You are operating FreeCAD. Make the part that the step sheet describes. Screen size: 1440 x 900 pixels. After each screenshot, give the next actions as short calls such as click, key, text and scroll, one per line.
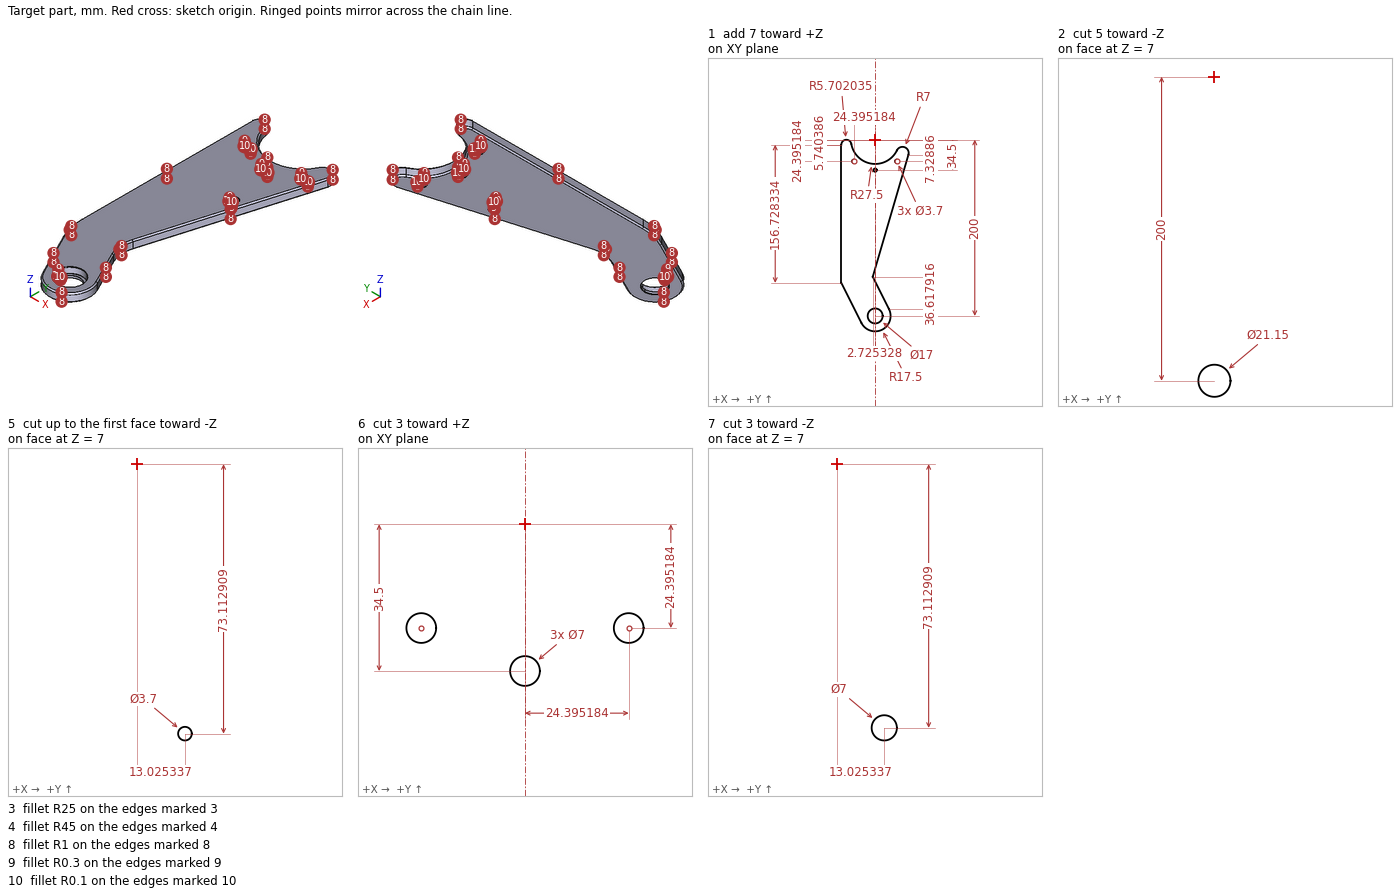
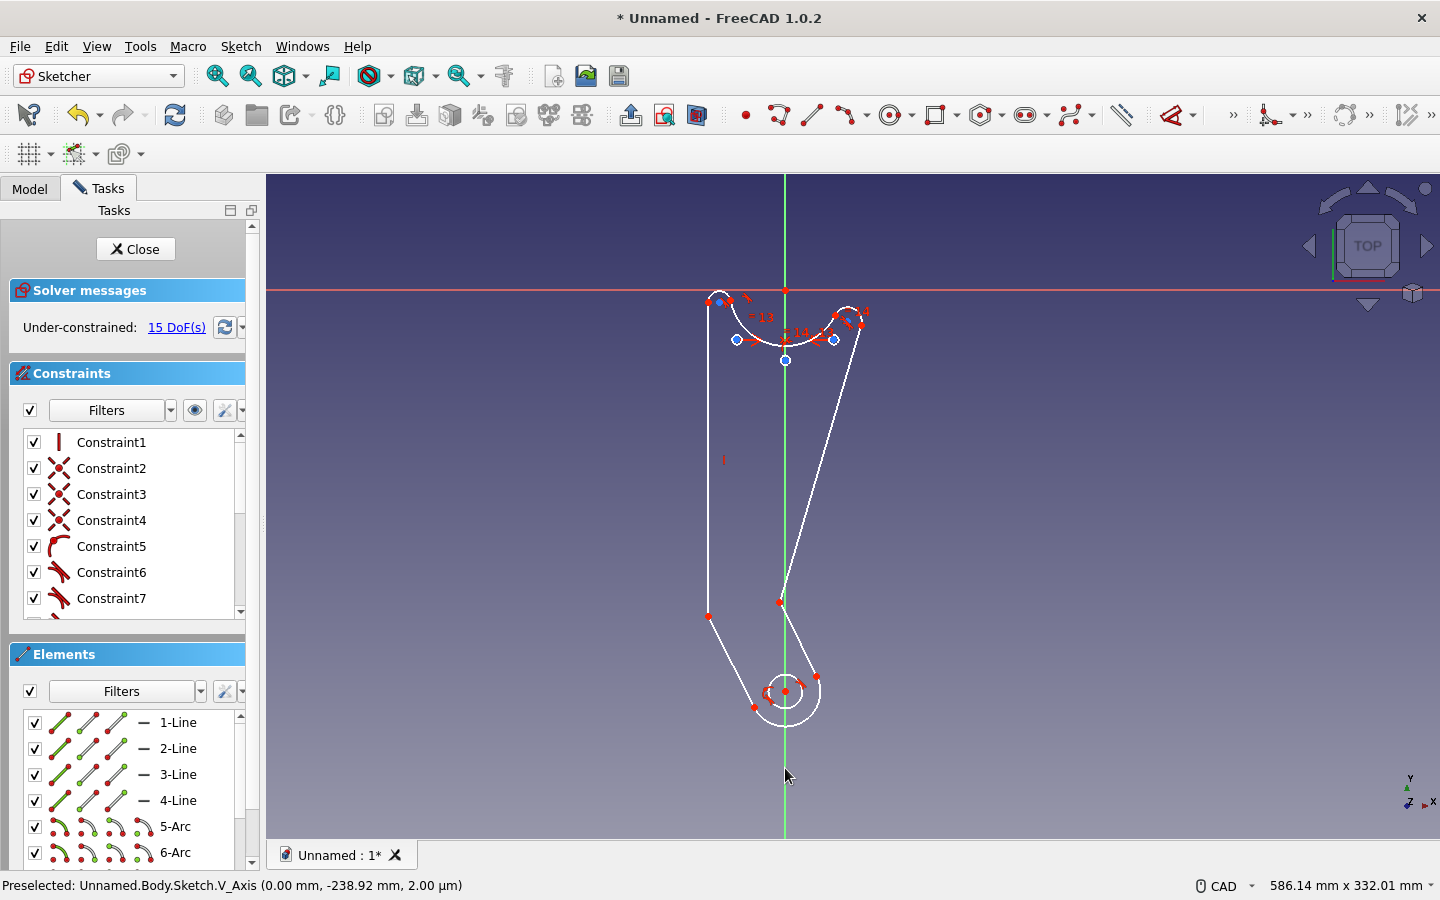
key(d)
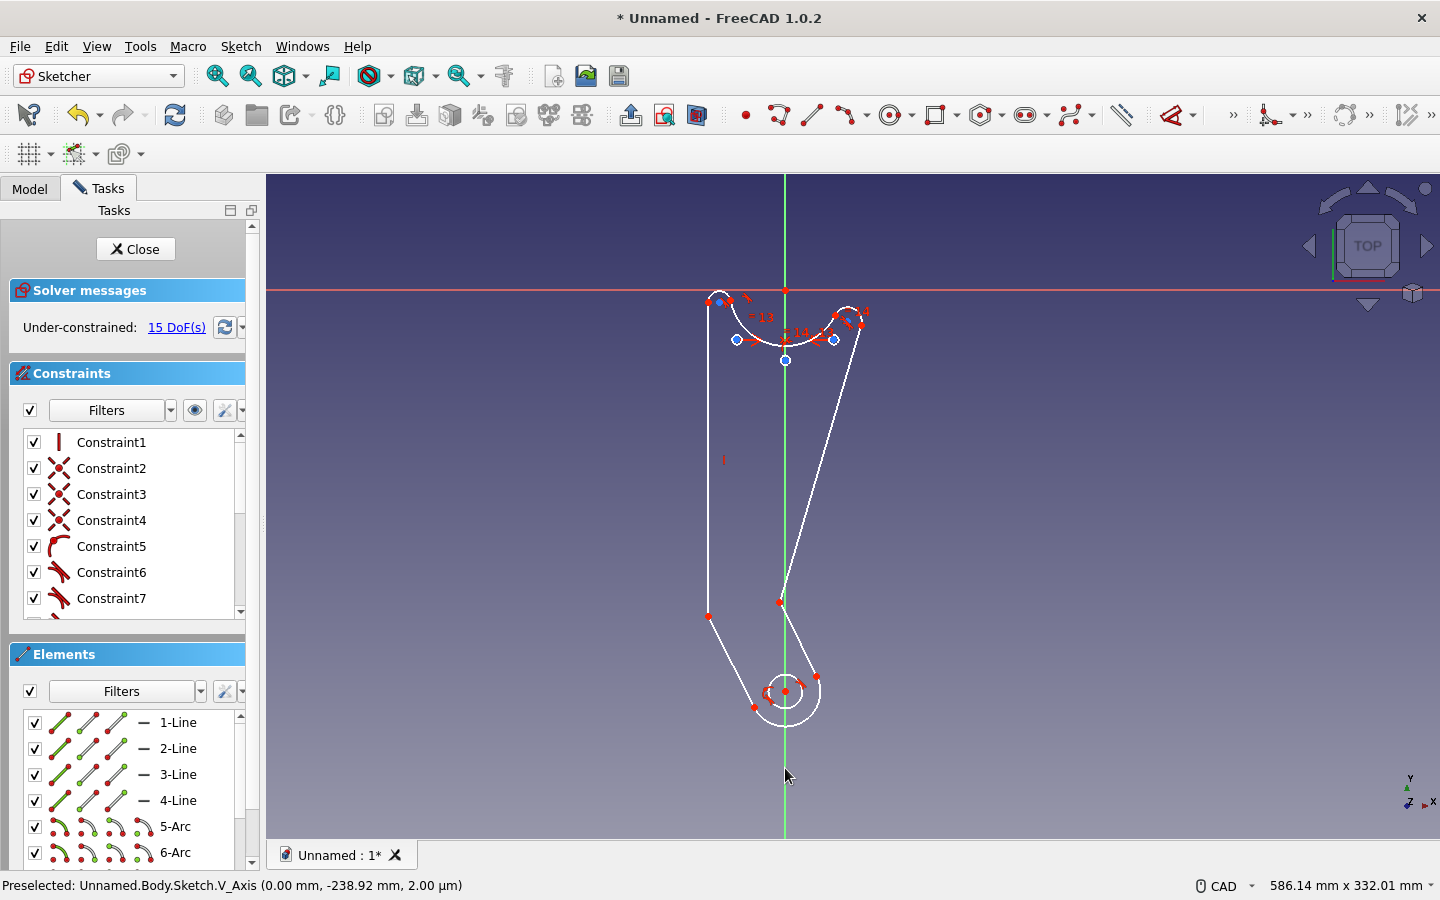
click(816, 708)
click(844, 723)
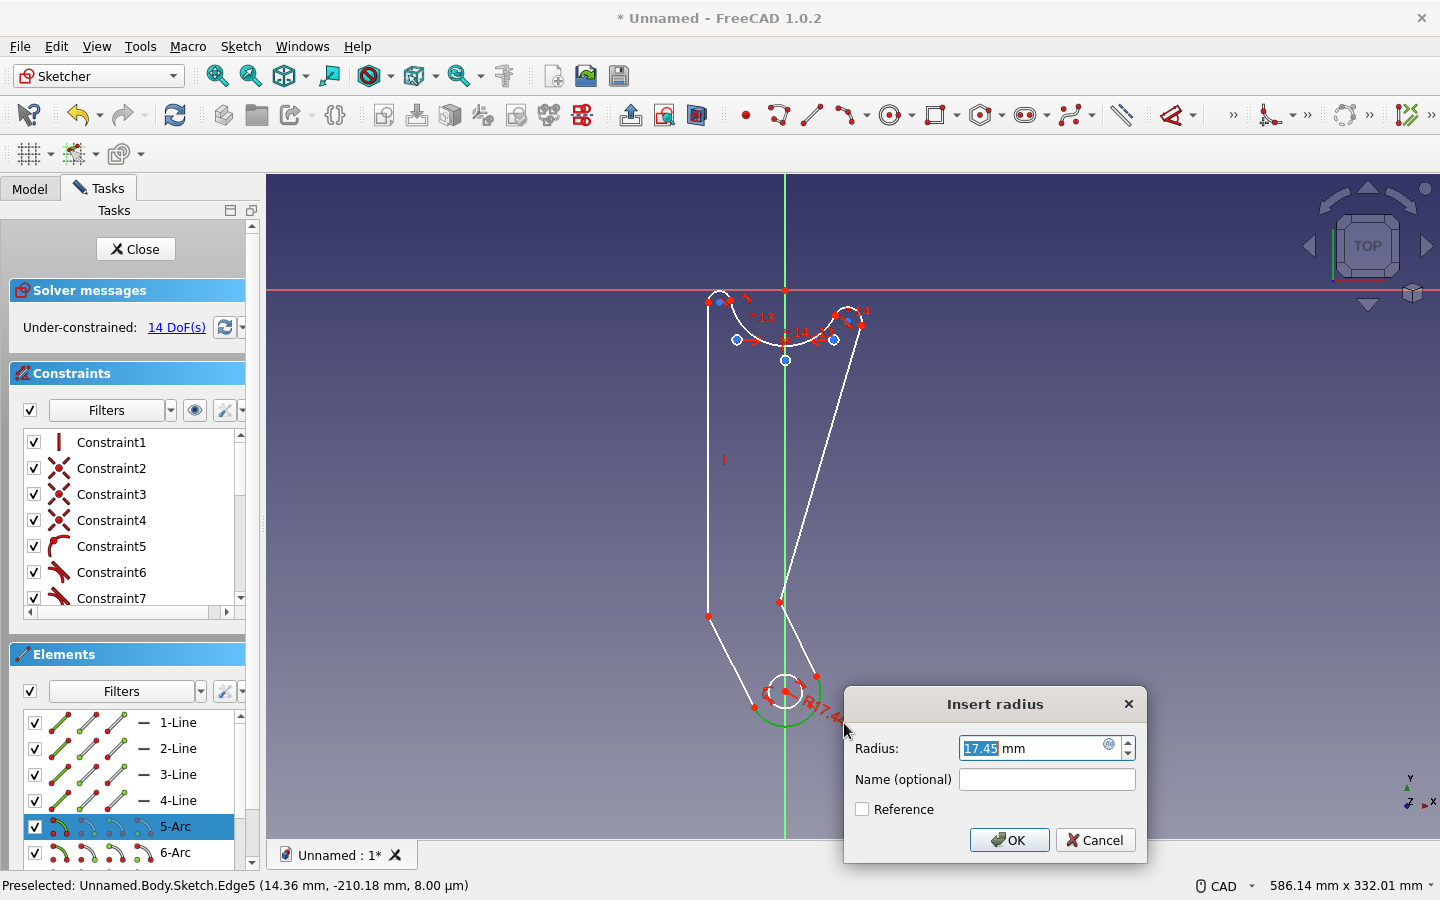
text(17.5)
key(Return)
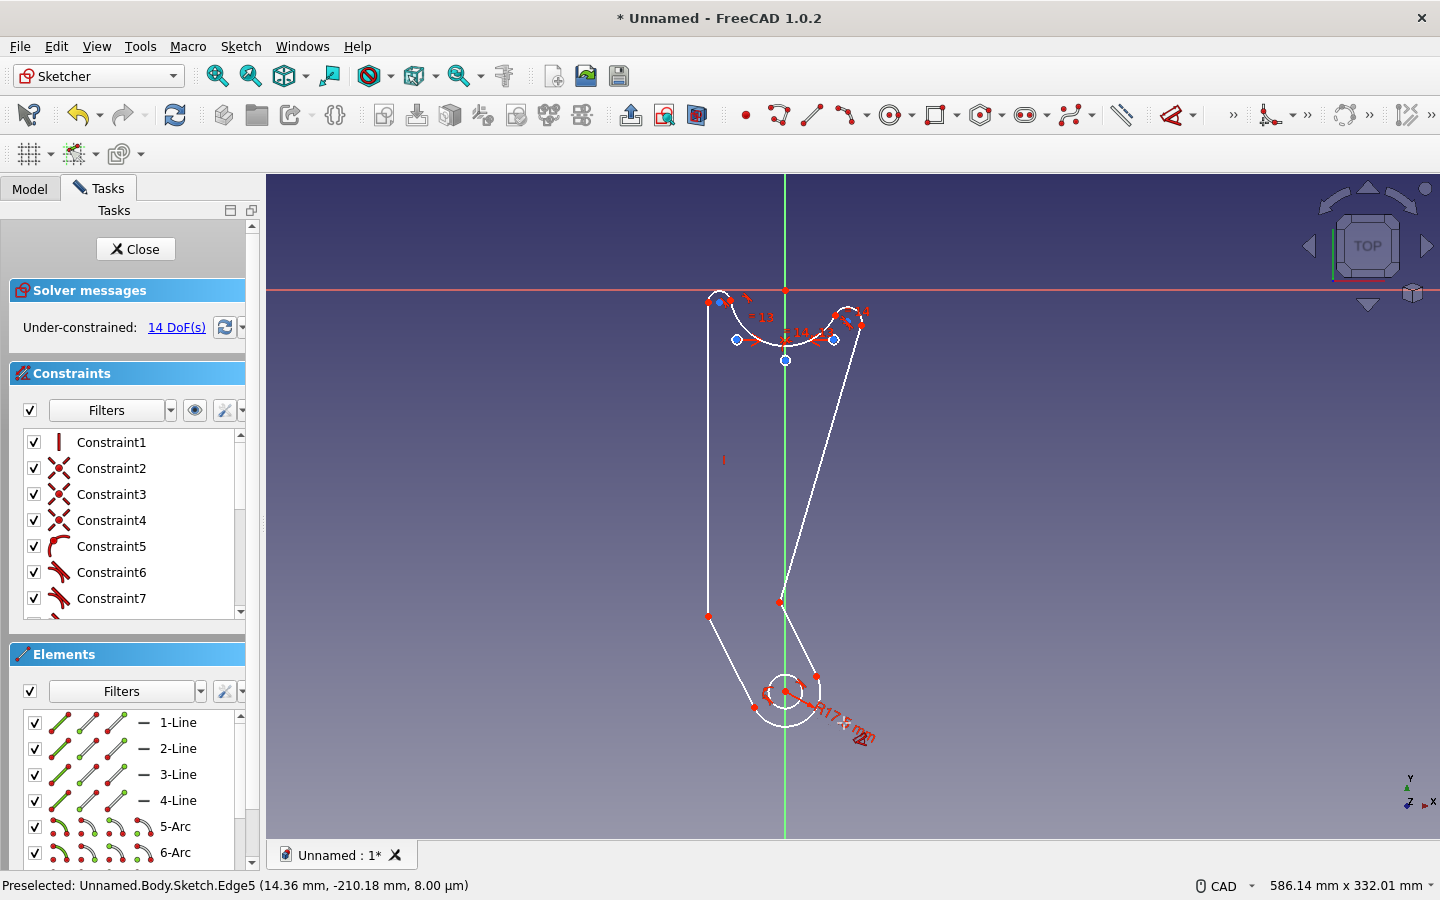
scroll(859, 313, up, 6)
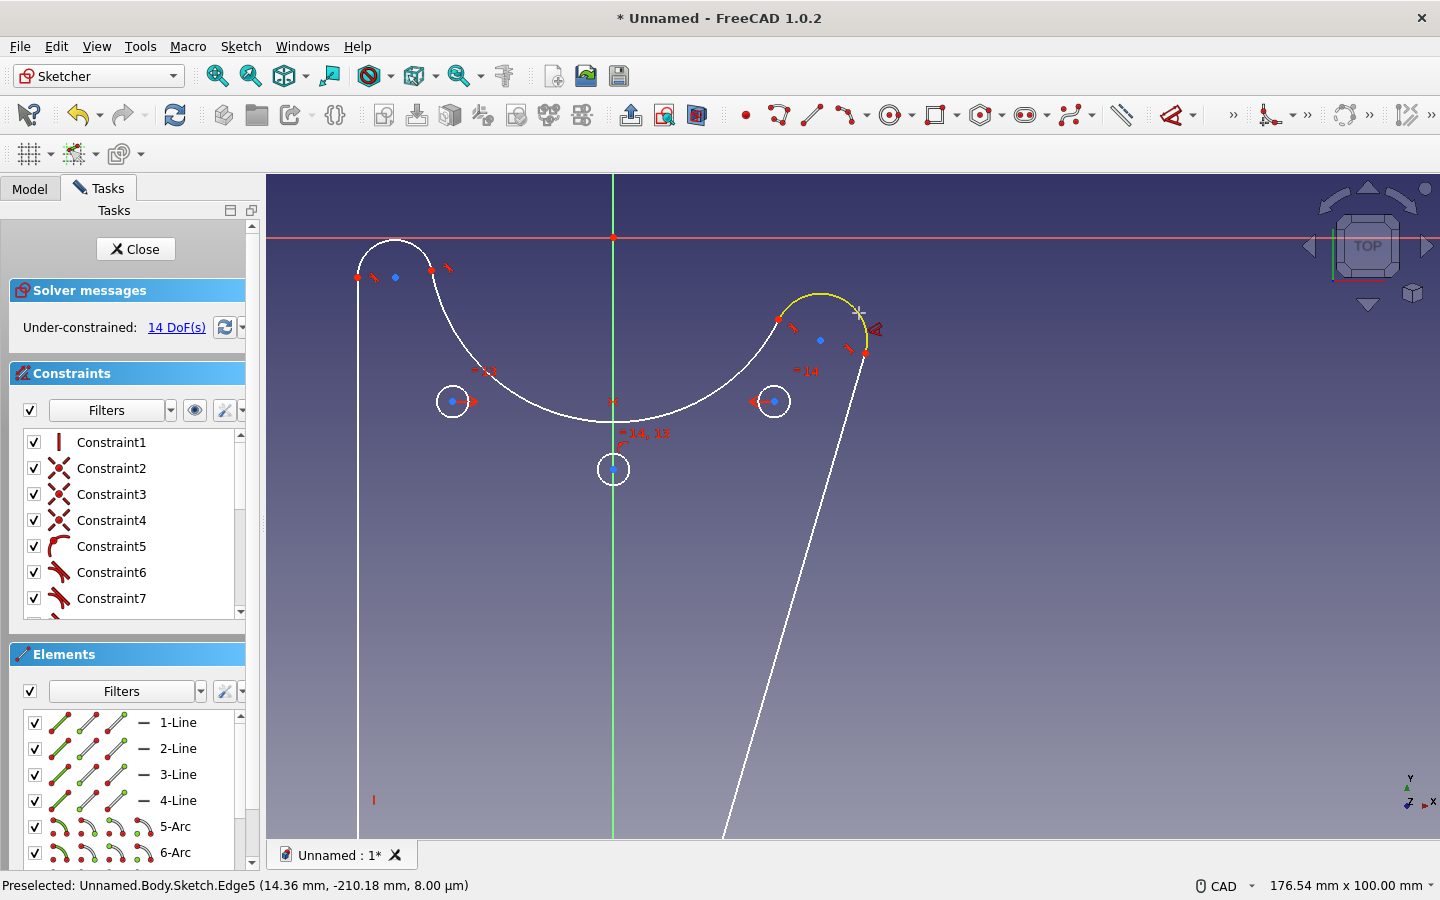
click(859, 314)
click(885, 296)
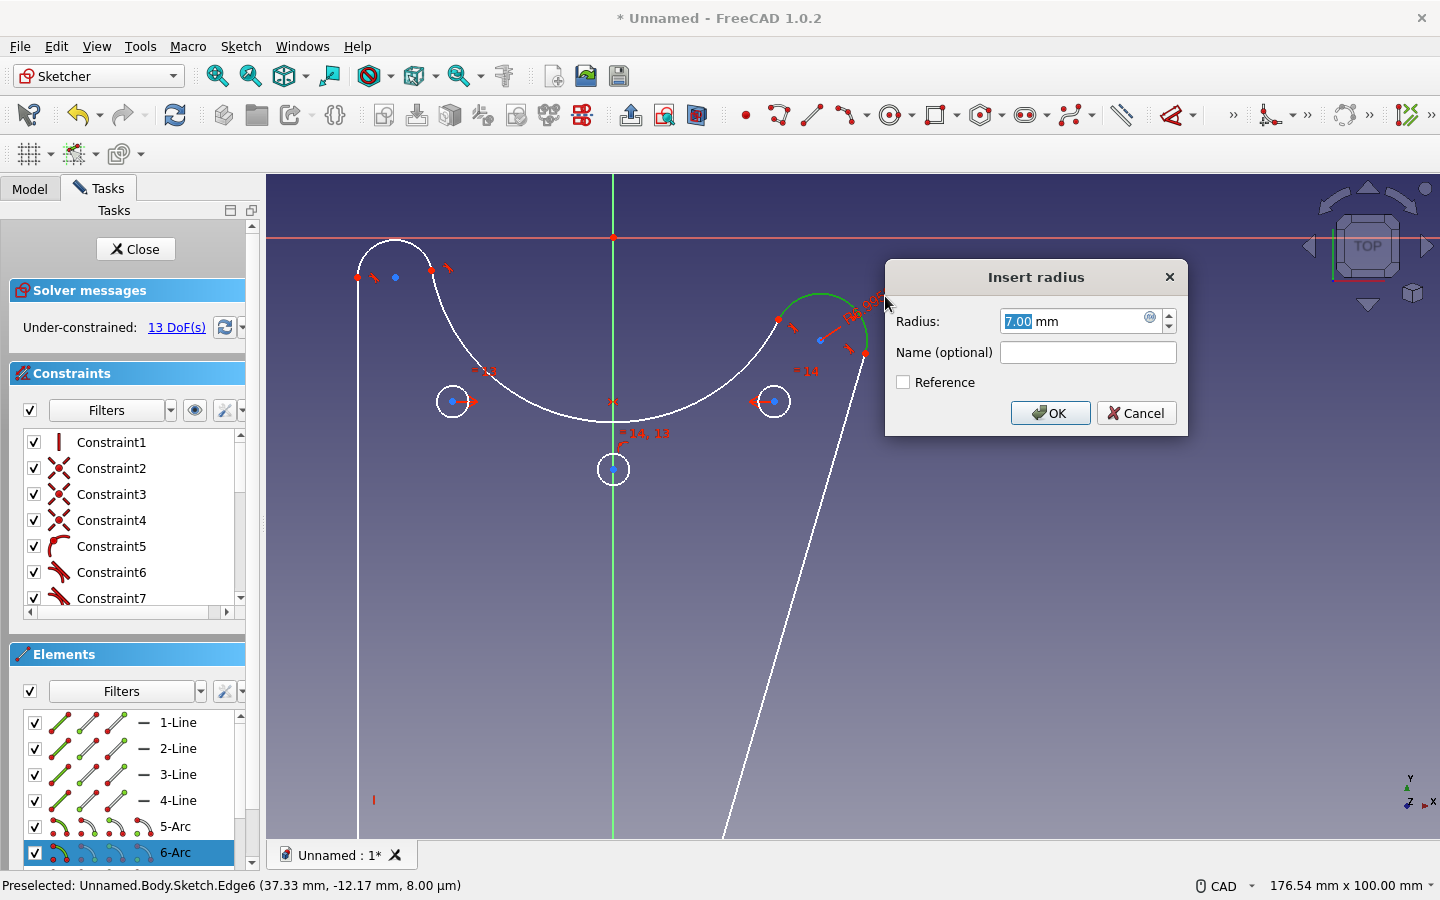
text(7)
key(Return)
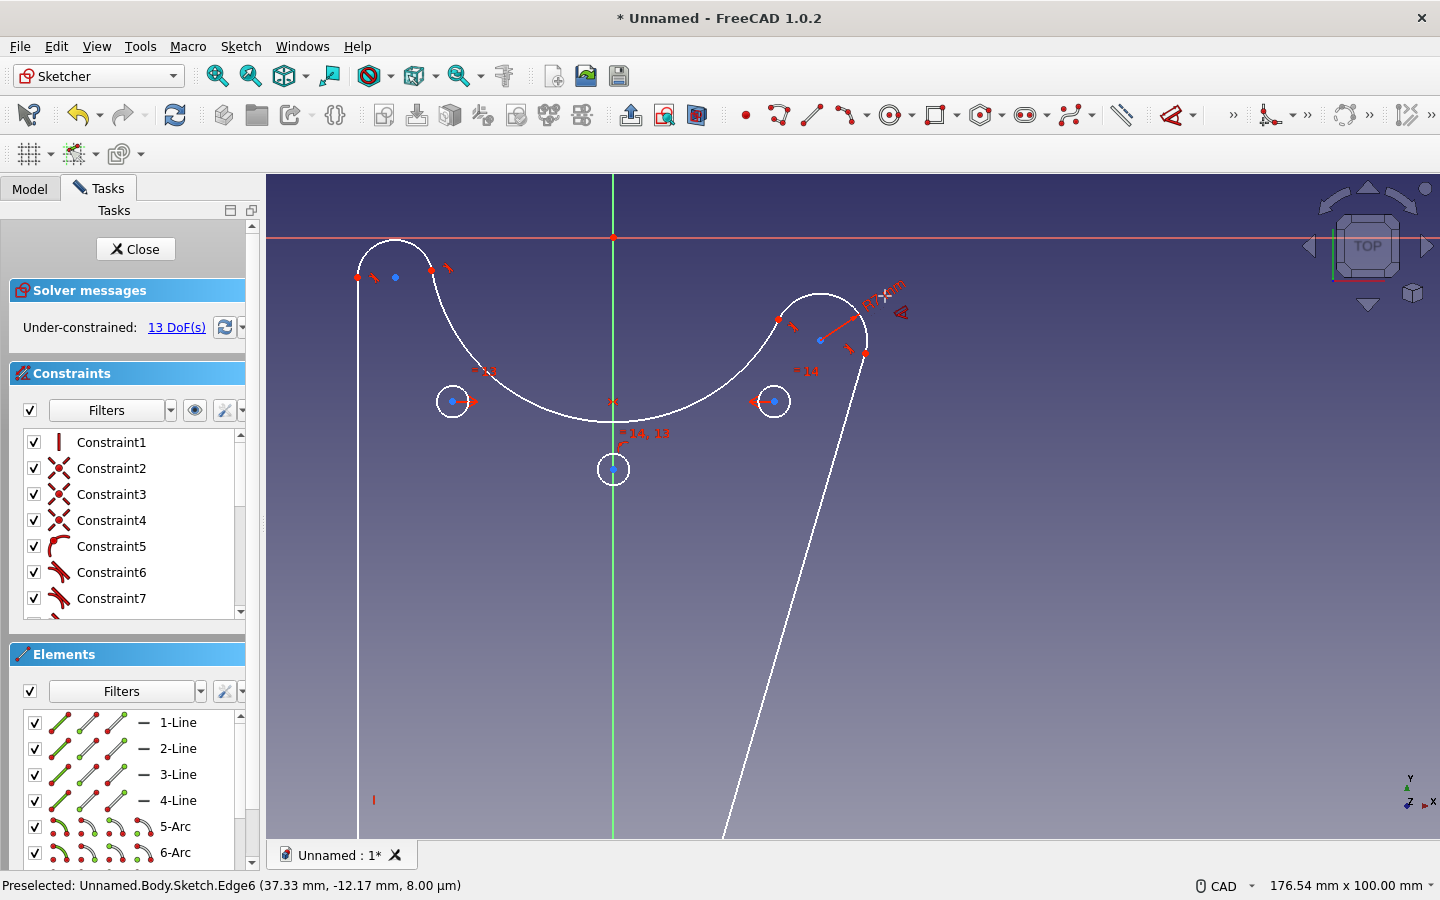
click(503, 386)
click(484, 412)